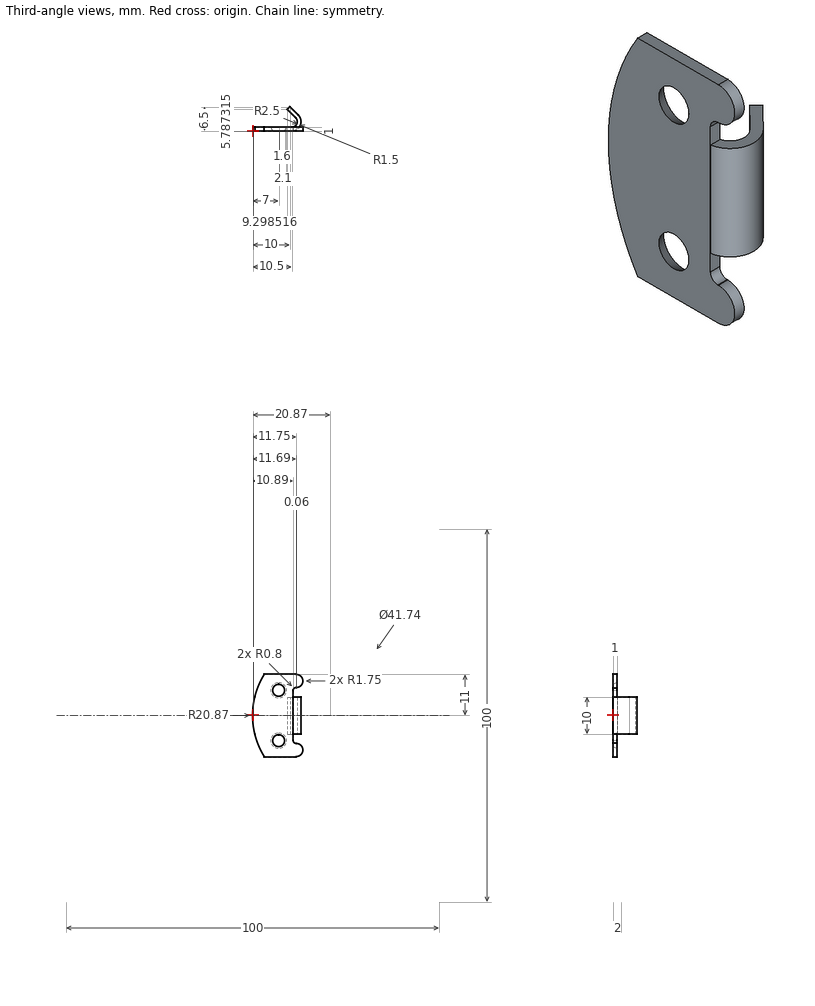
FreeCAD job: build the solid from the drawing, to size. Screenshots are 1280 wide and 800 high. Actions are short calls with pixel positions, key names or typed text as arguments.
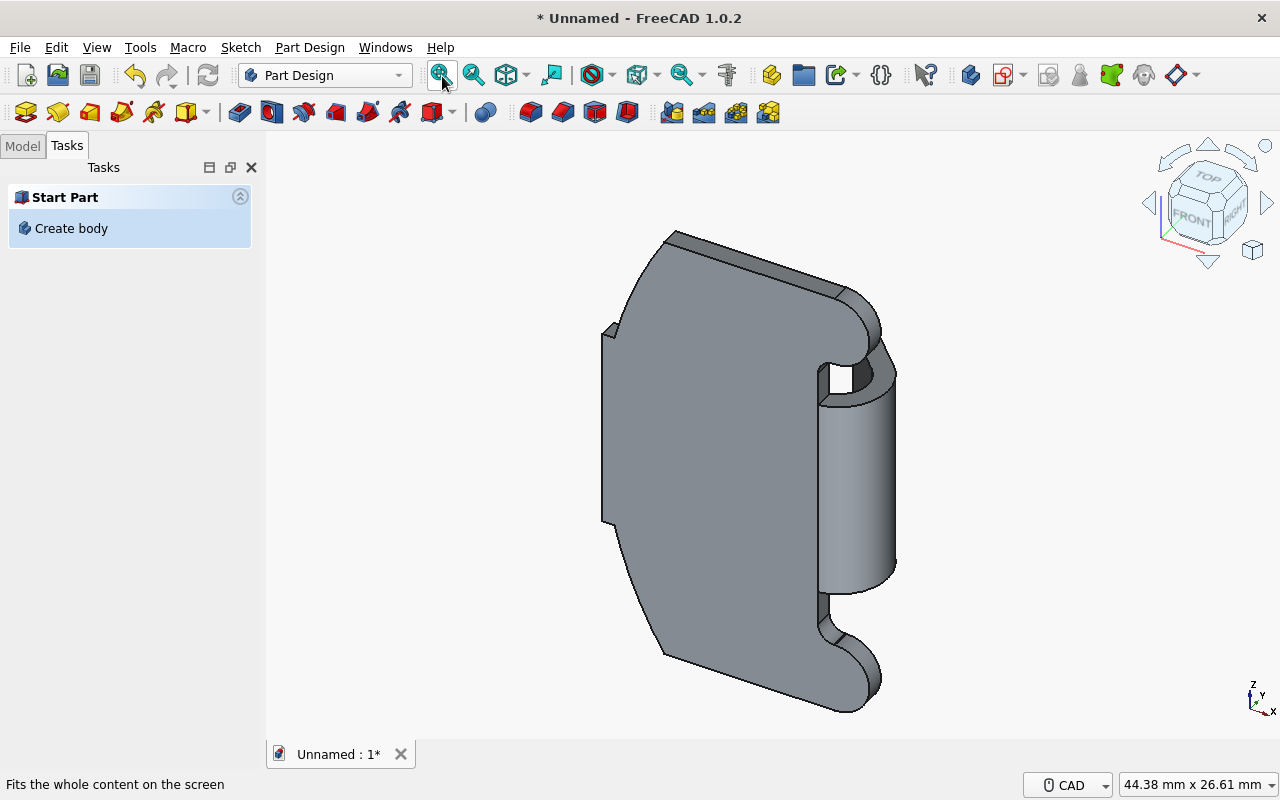
click(698, 458)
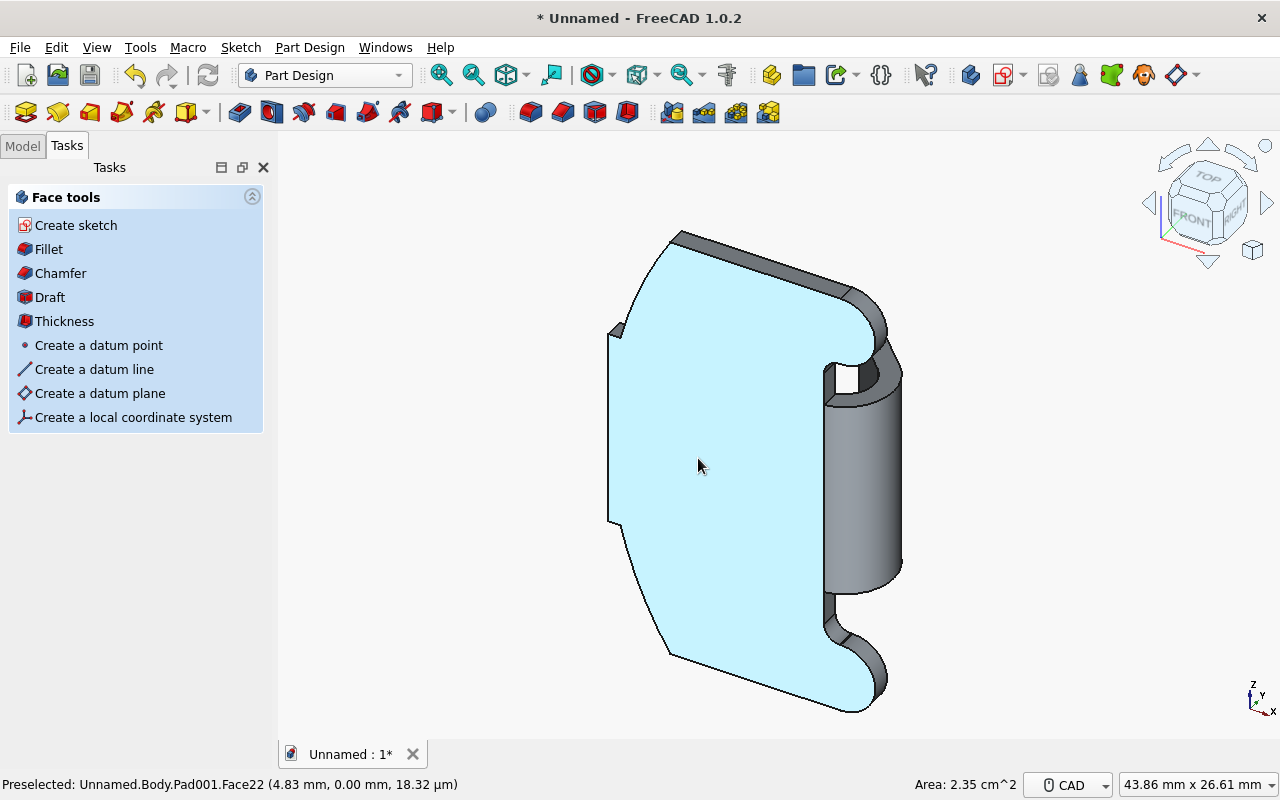
click(1004, 76)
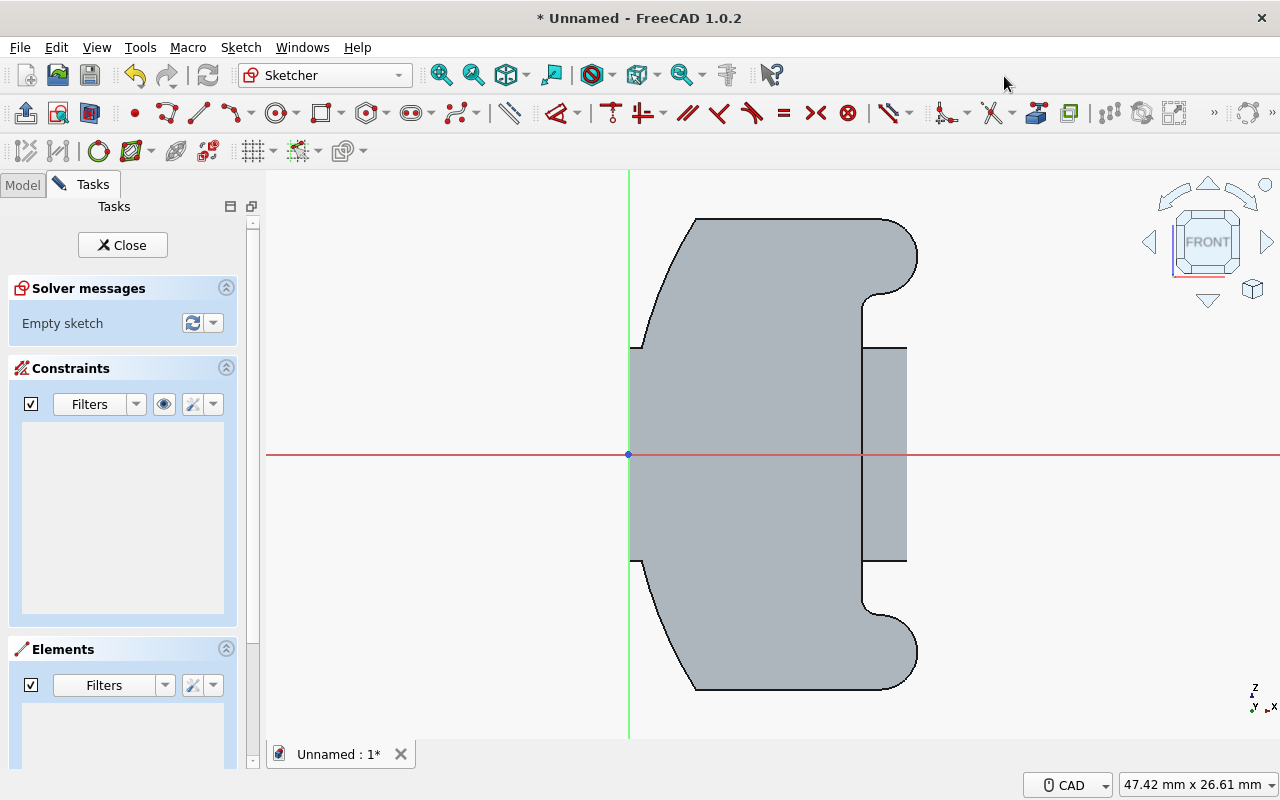
scroll(719, 454, down, 9)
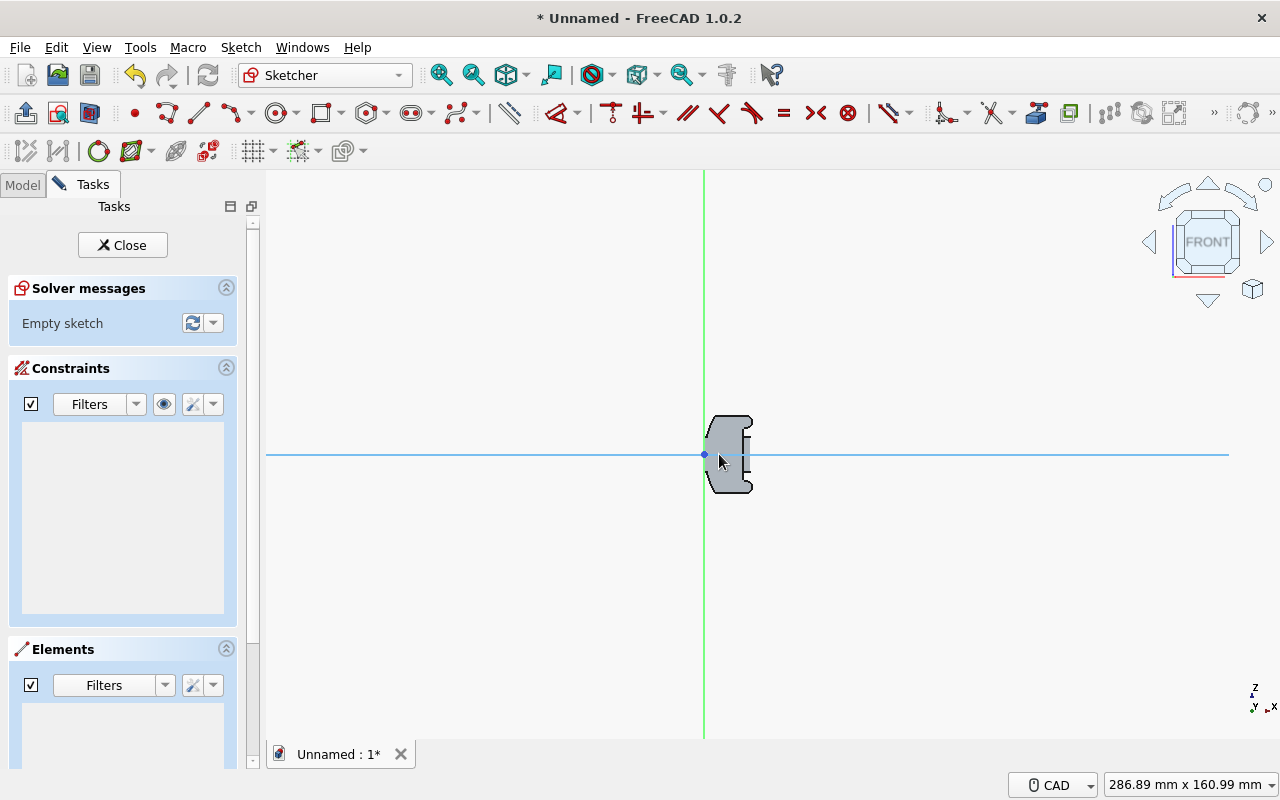
click(344, 114)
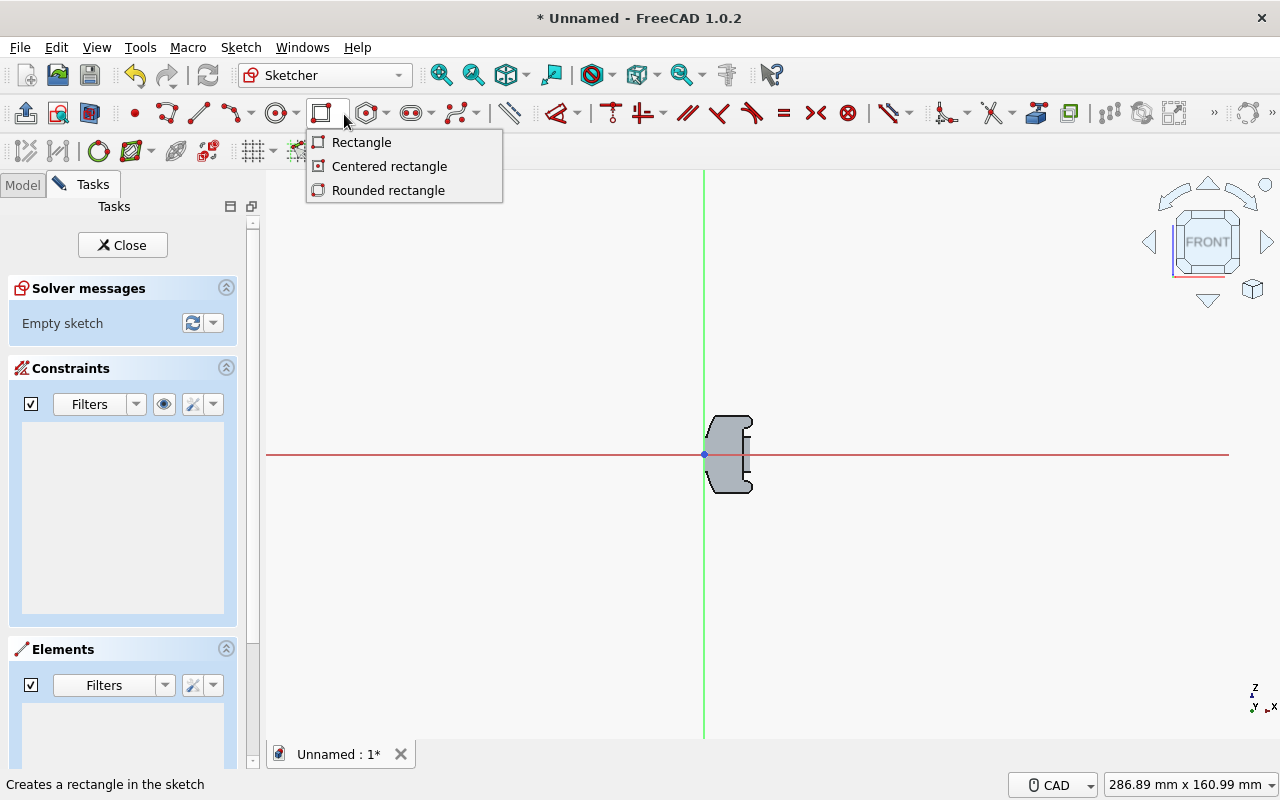
click(404, 166)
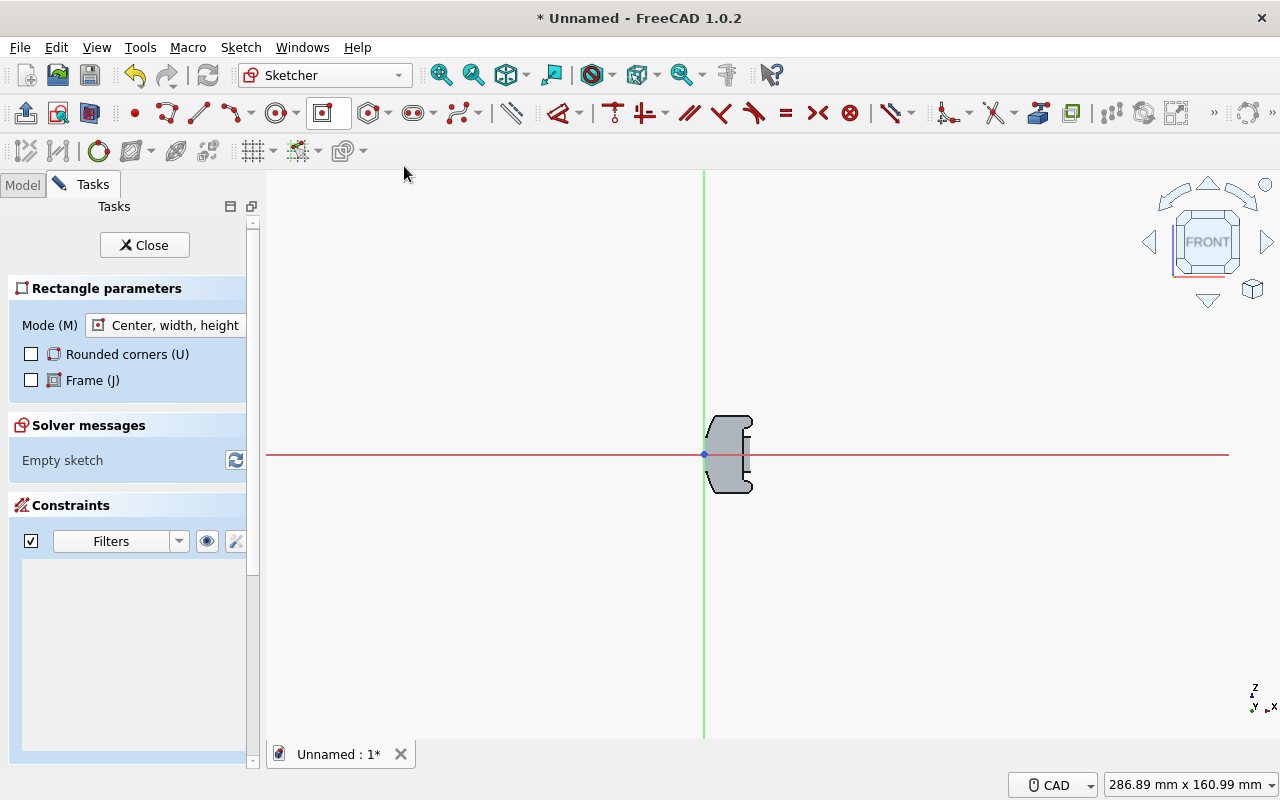
click(704, 455)
move(881, 278)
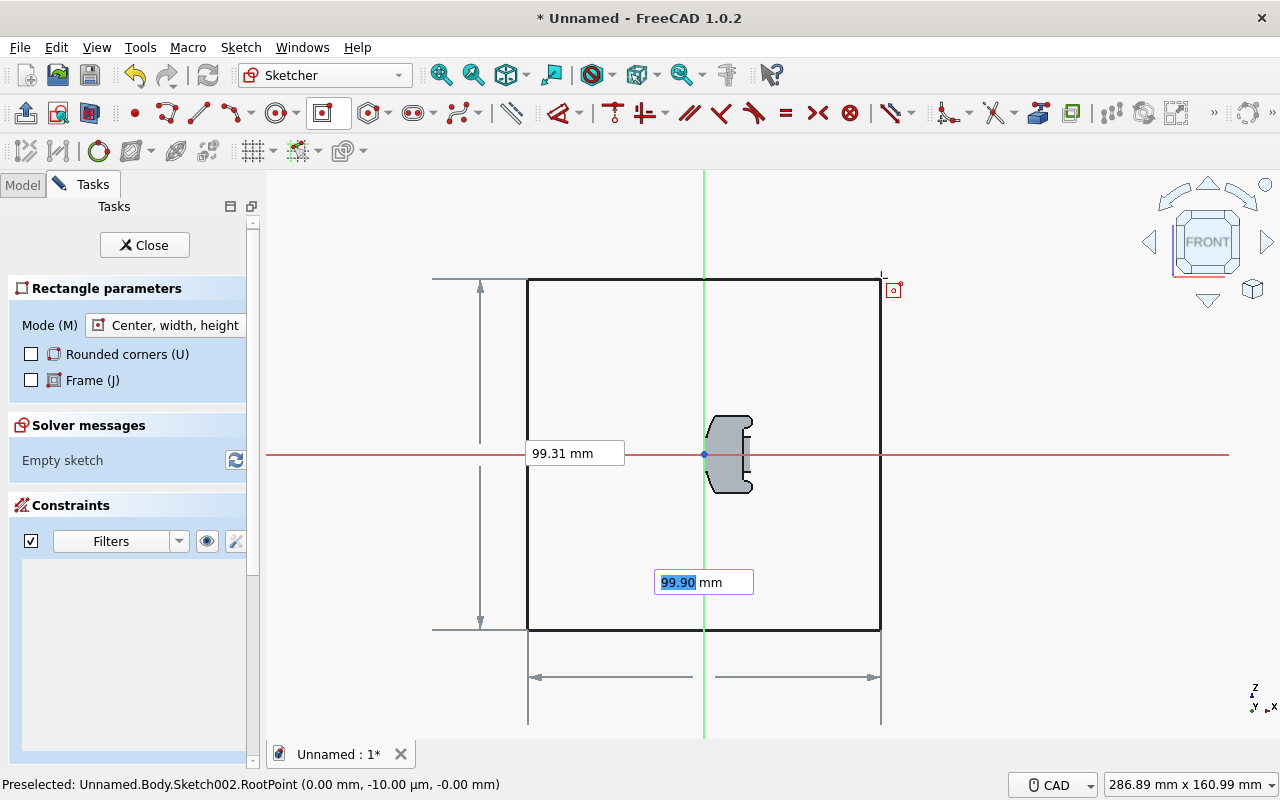
text(100)
key(Tab)
text(100)
key(Return)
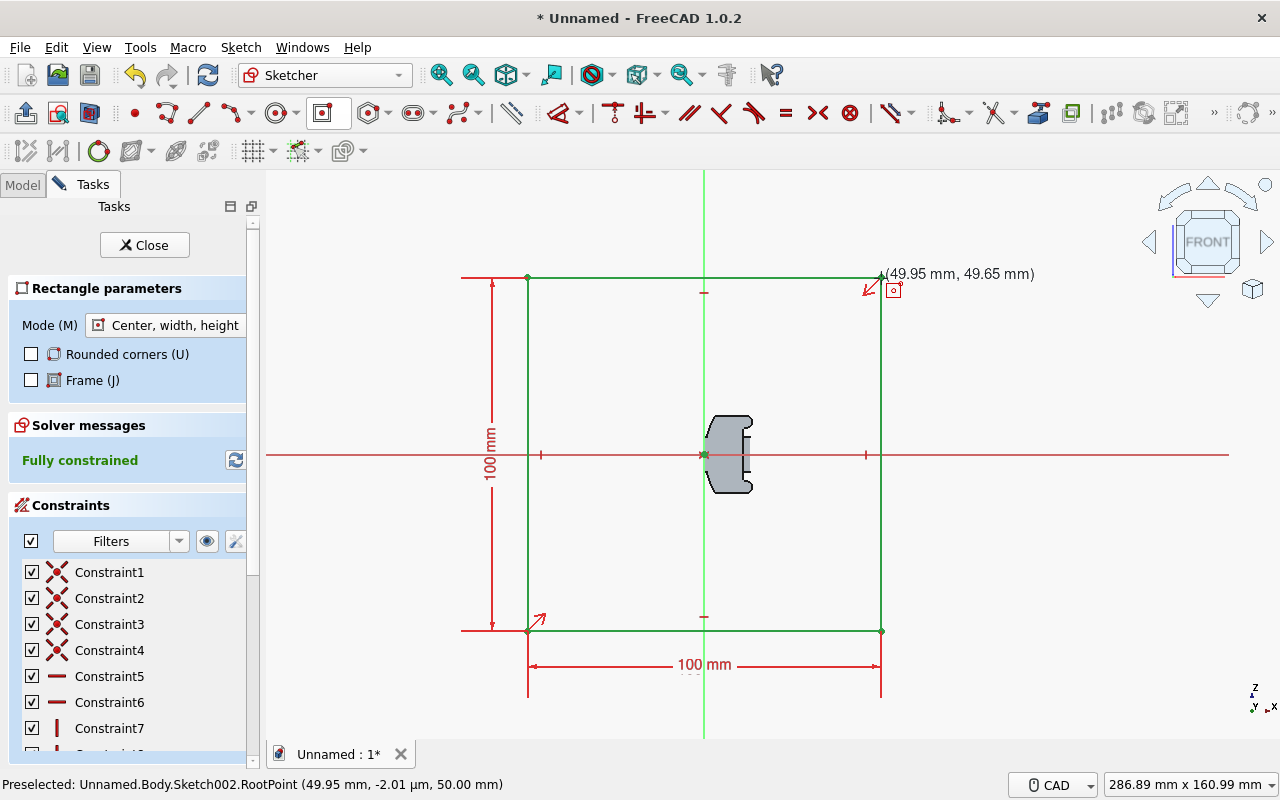
click(276, 114)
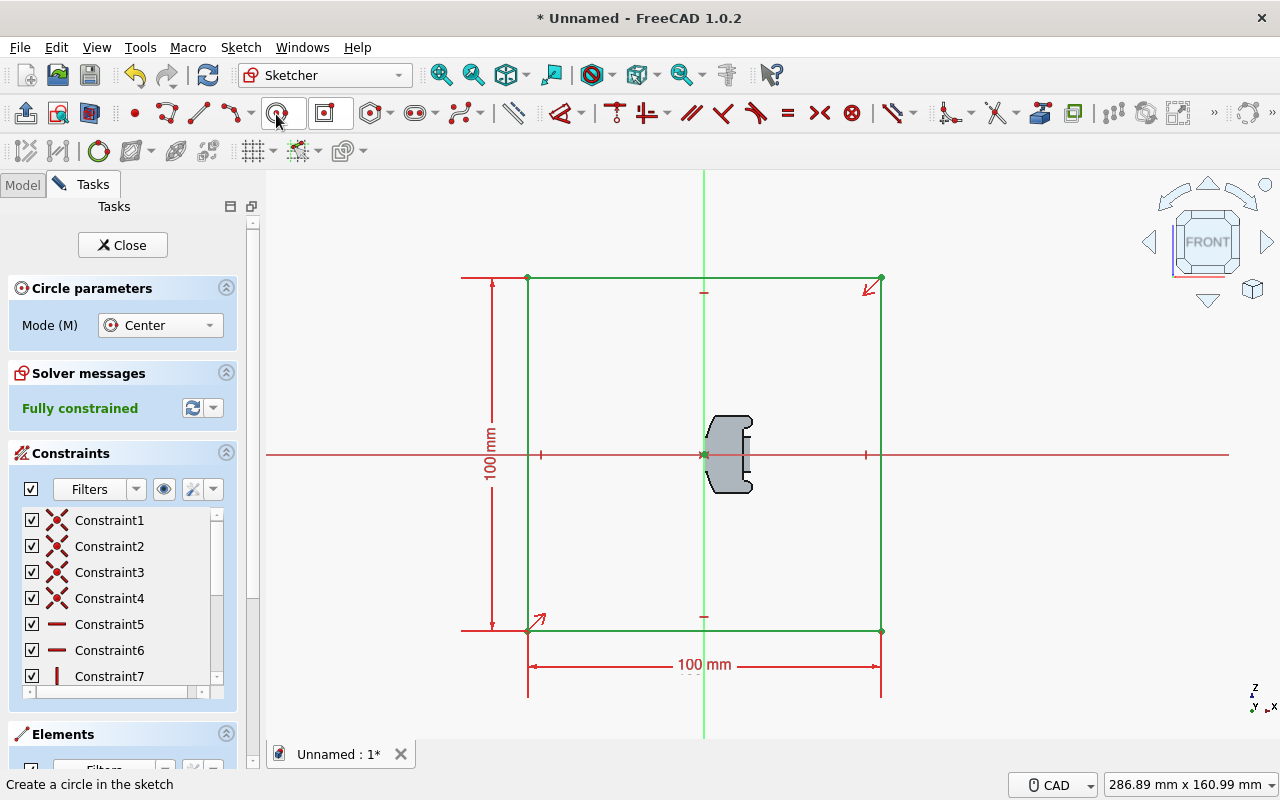
click(778, 455)
move(830, 402)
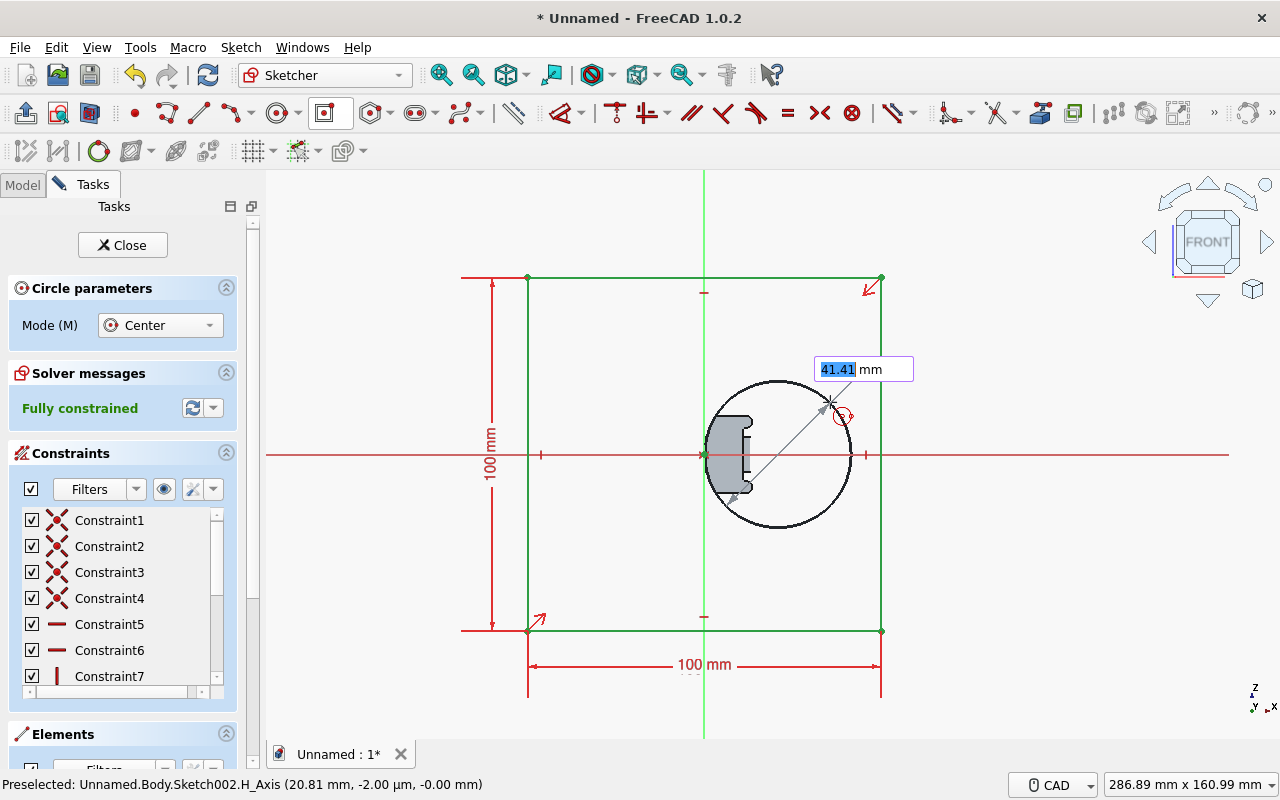
text(41.74)
key(Return)
key(Escape)